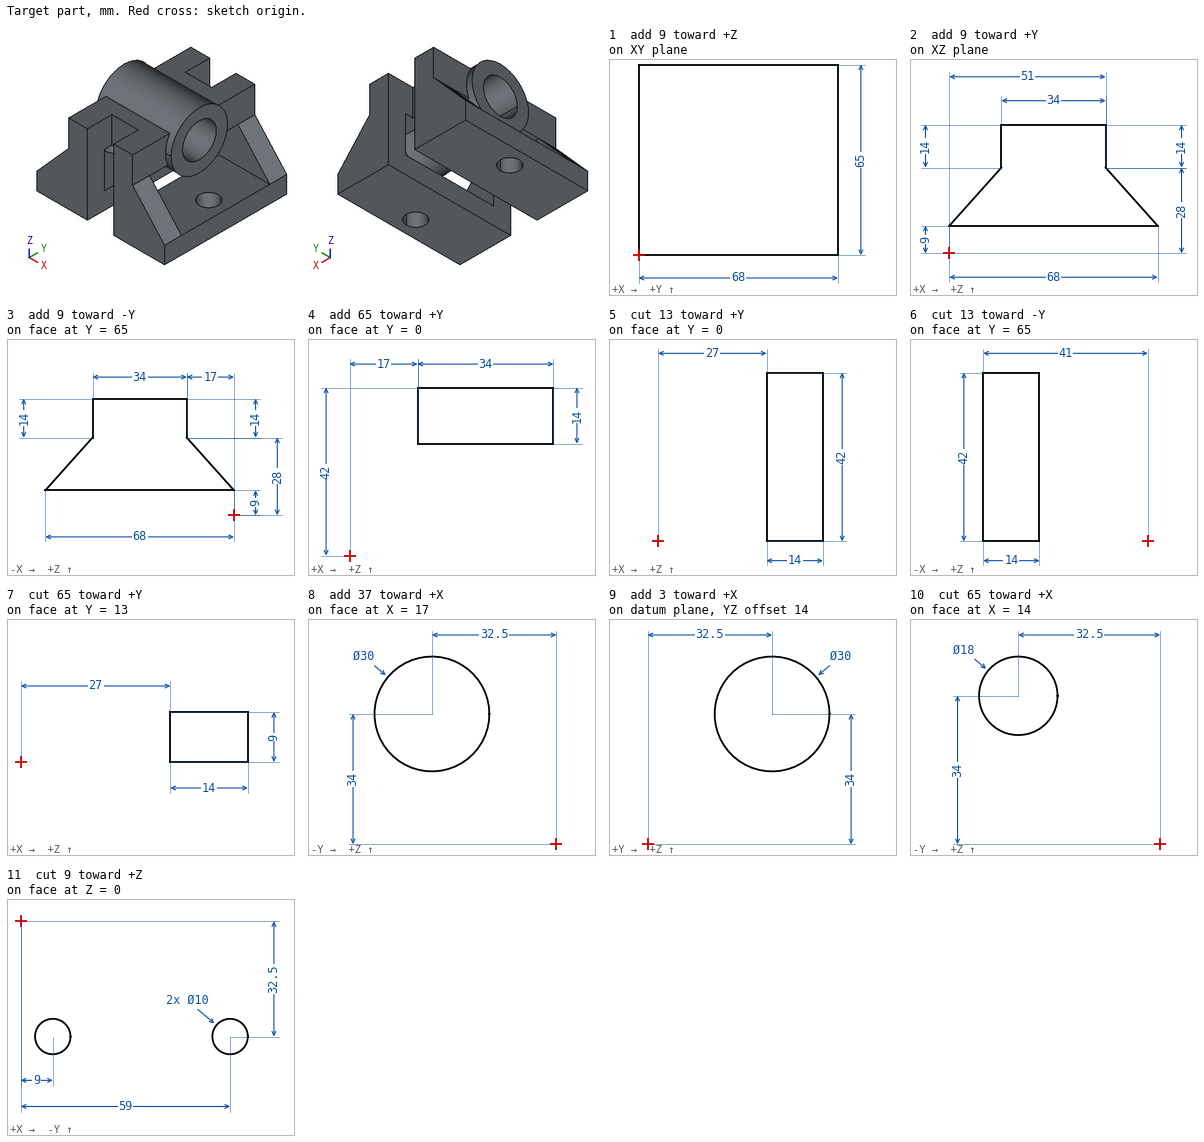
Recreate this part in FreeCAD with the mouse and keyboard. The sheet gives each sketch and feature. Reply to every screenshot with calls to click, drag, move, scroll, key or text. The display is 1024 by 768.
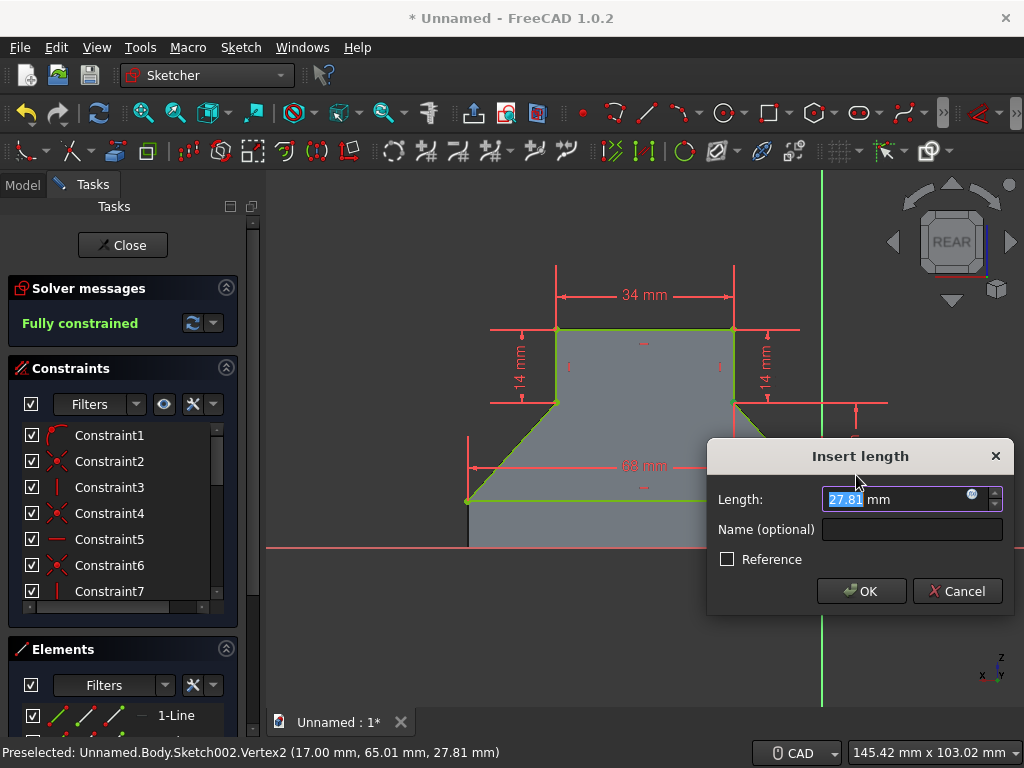
text(28)
key(Return)
key(Escape)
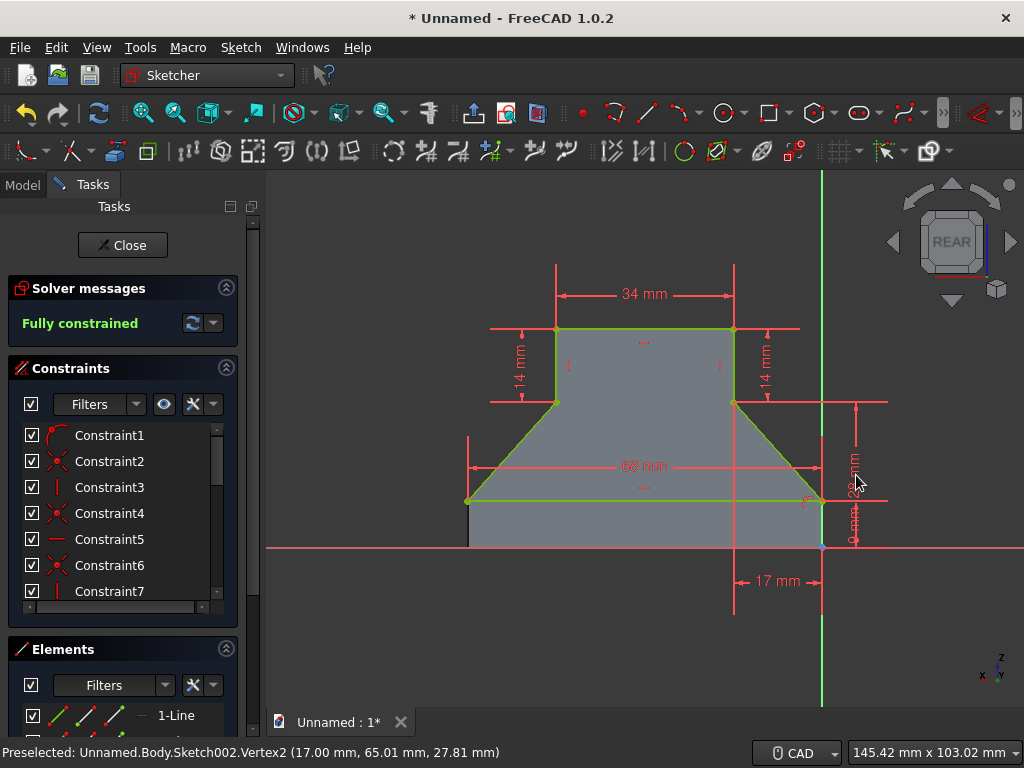
click(123, 245)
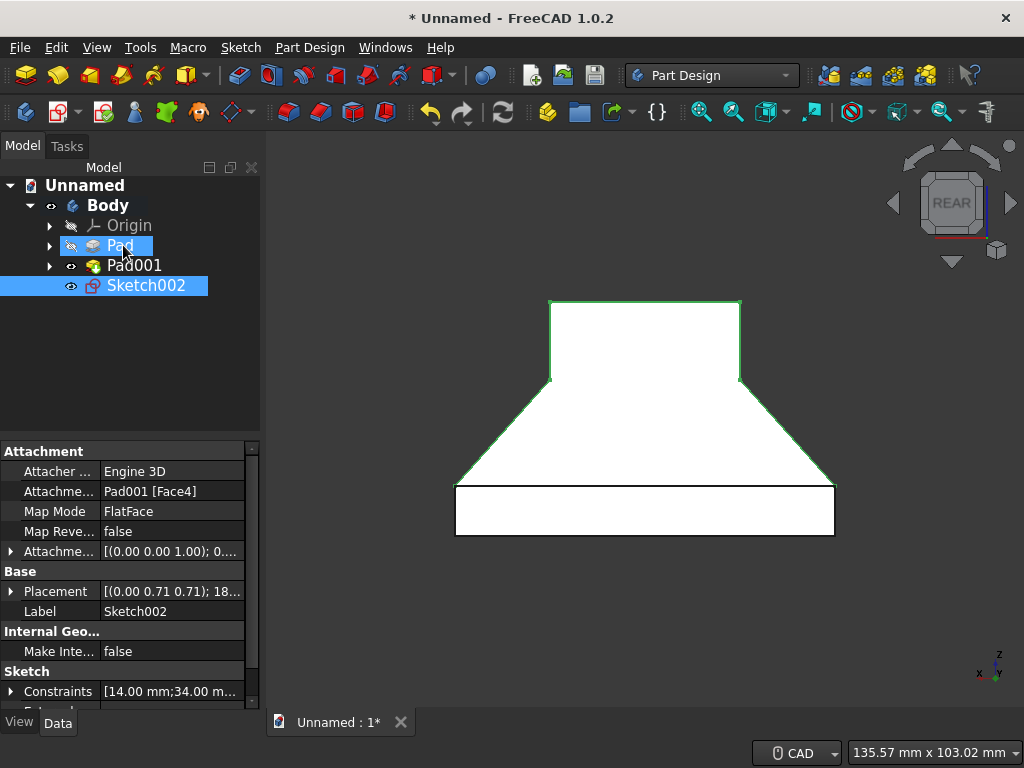
click(26, 76)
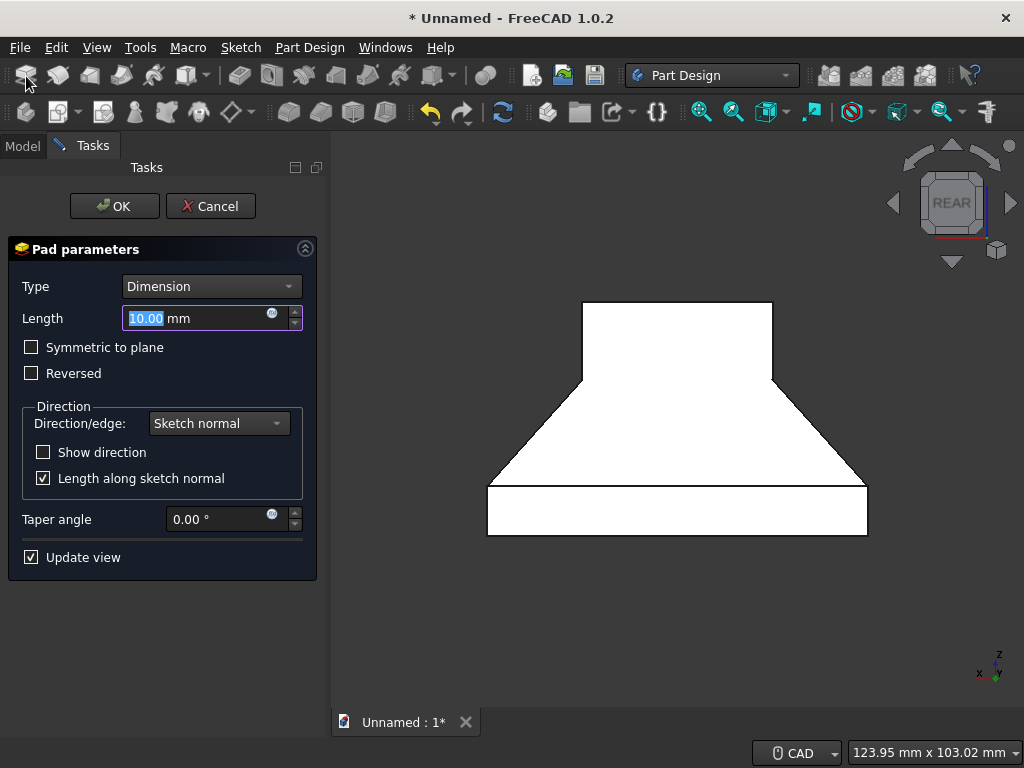
text(9)
key(Tab)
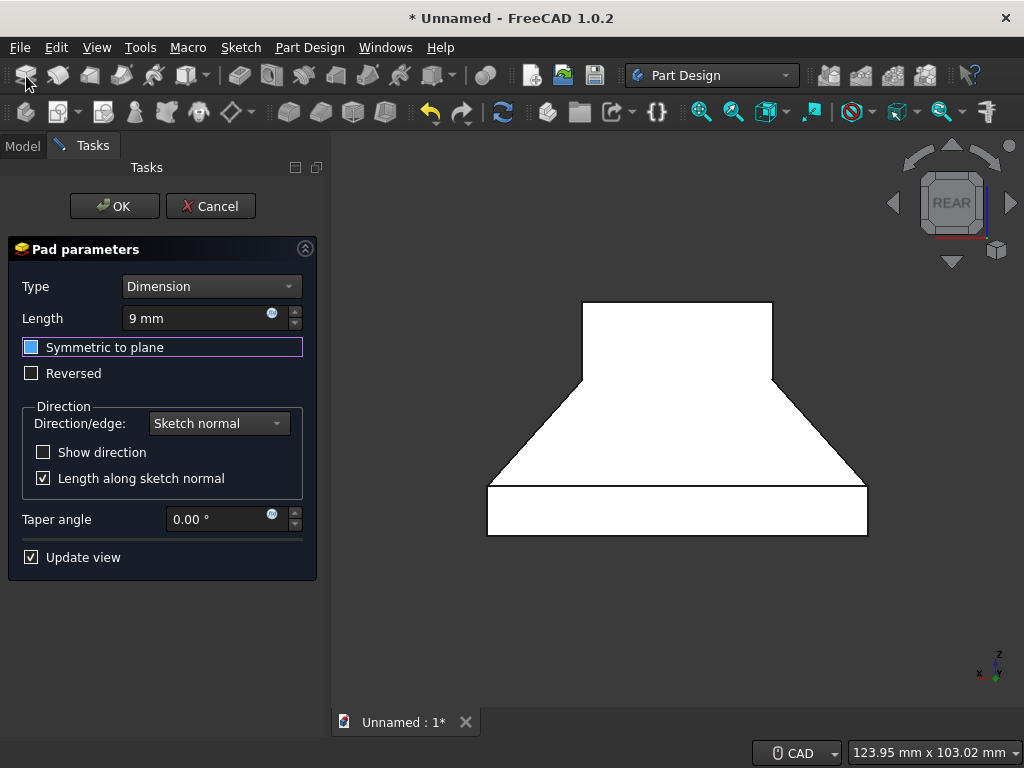
click(30, 373)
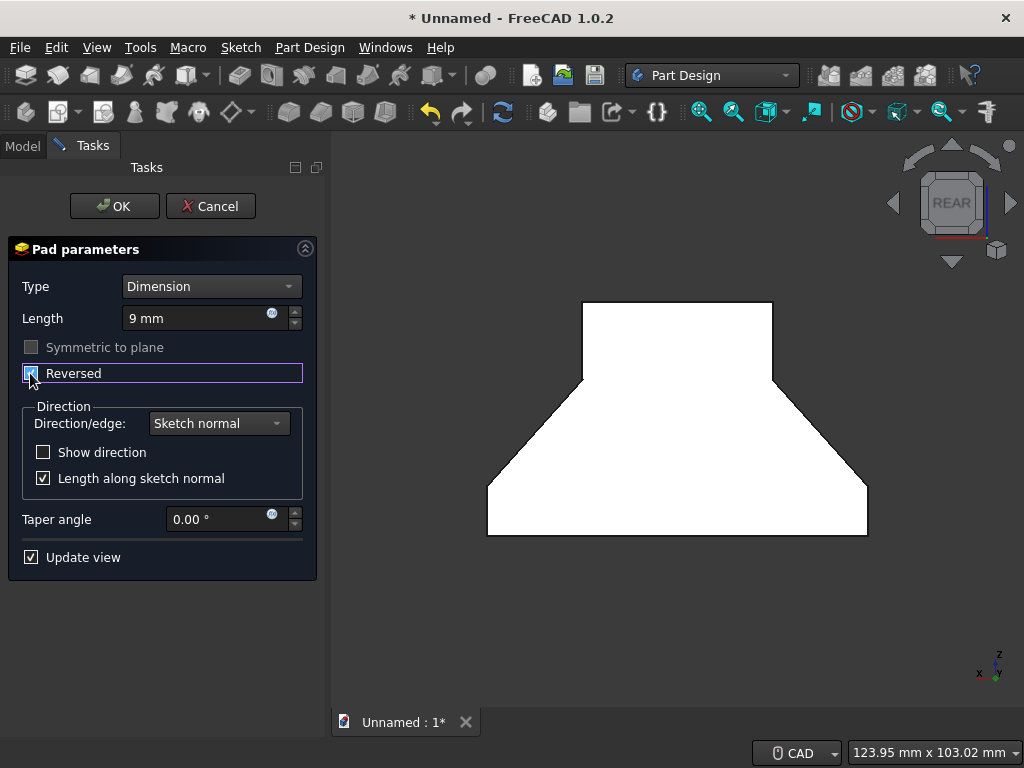
click(115, 206)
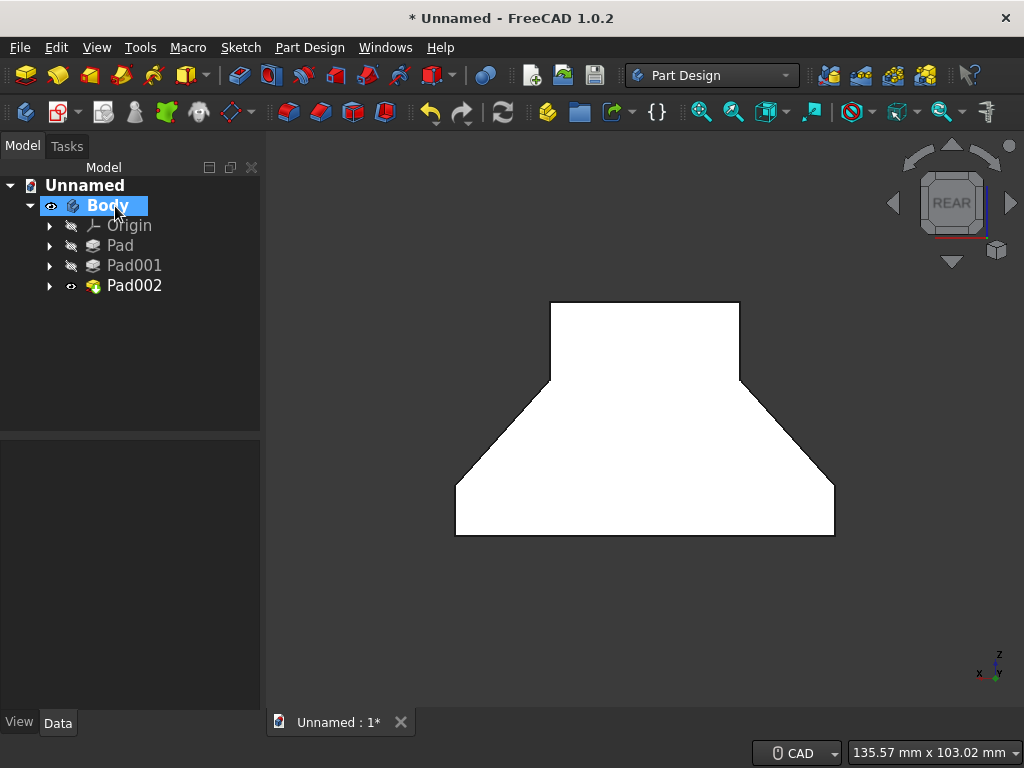
key(0)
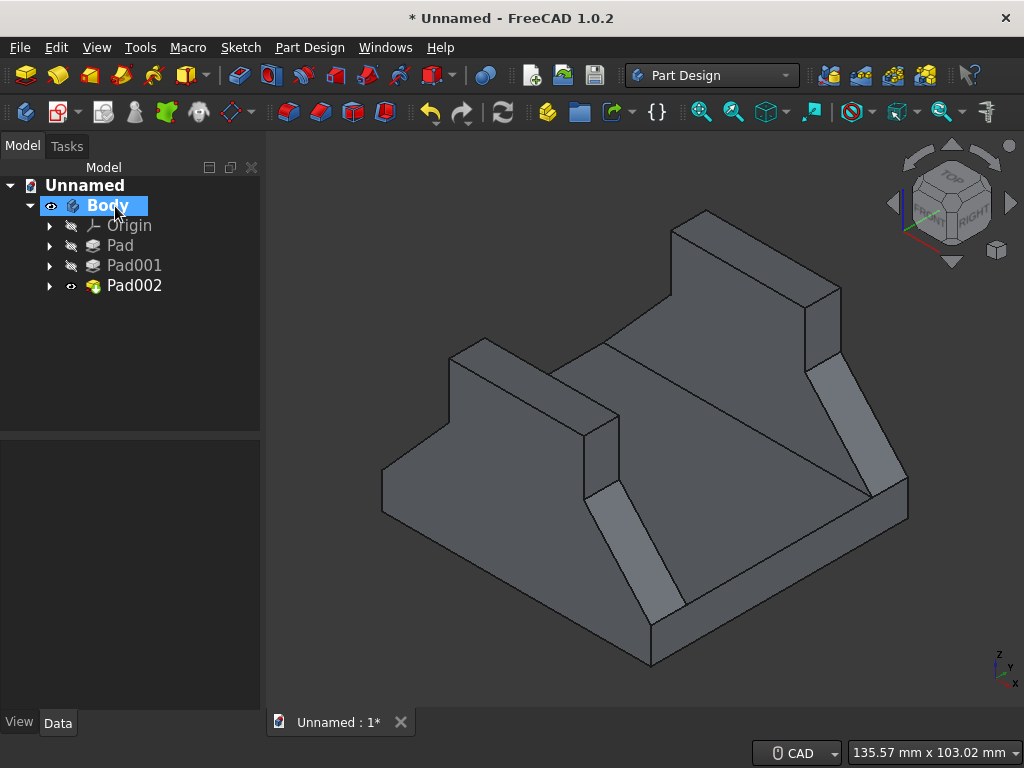
click(517, 492)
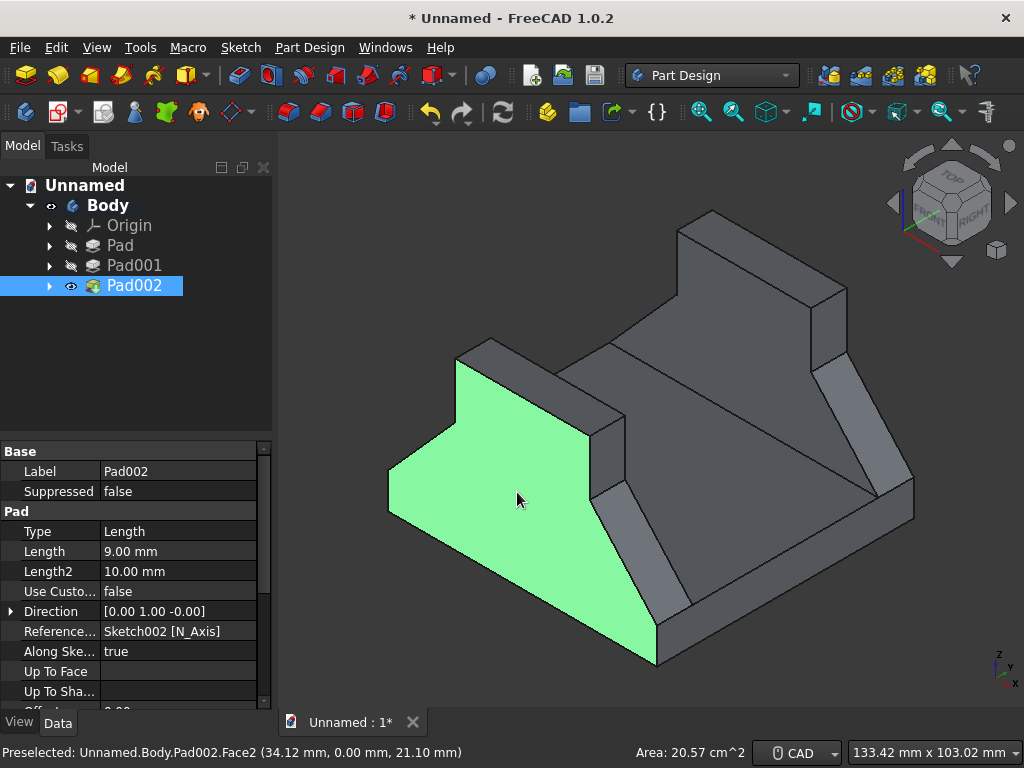
click(58, 112)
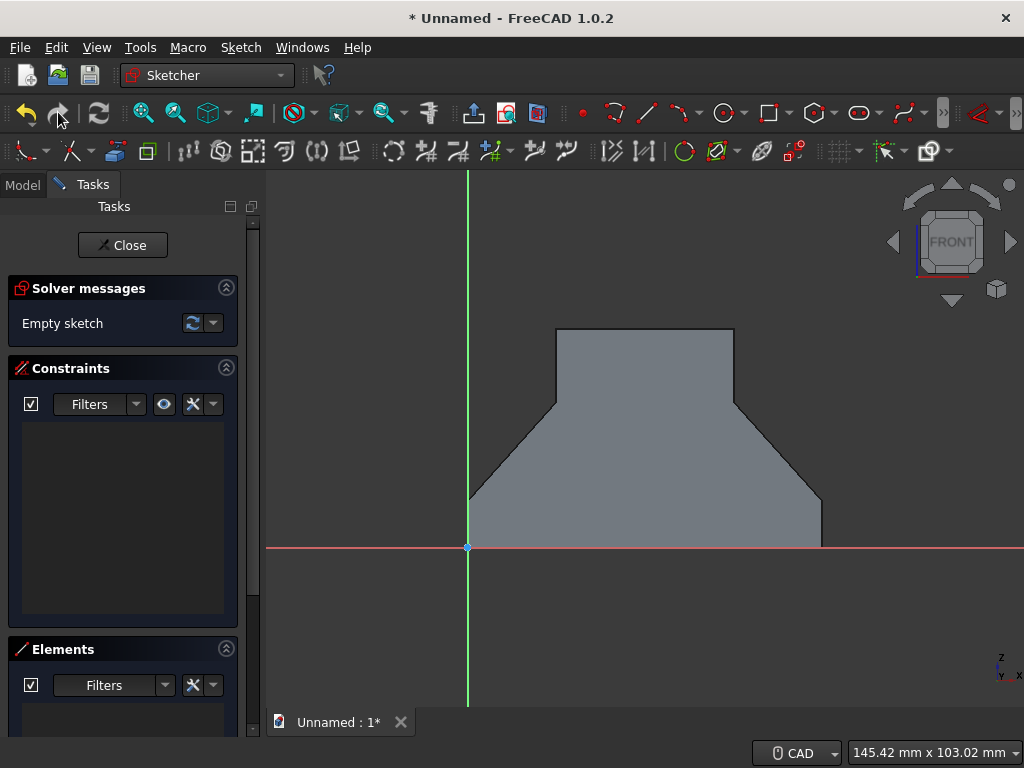
scroll(650, 439, up, 2)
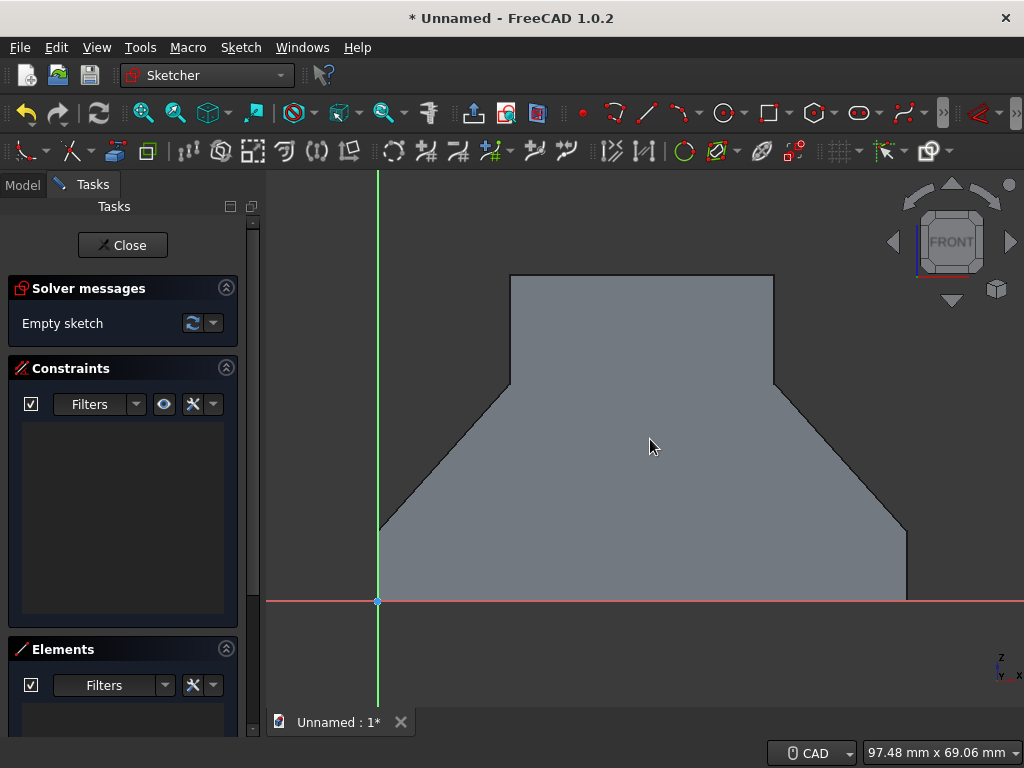
click(770, 114)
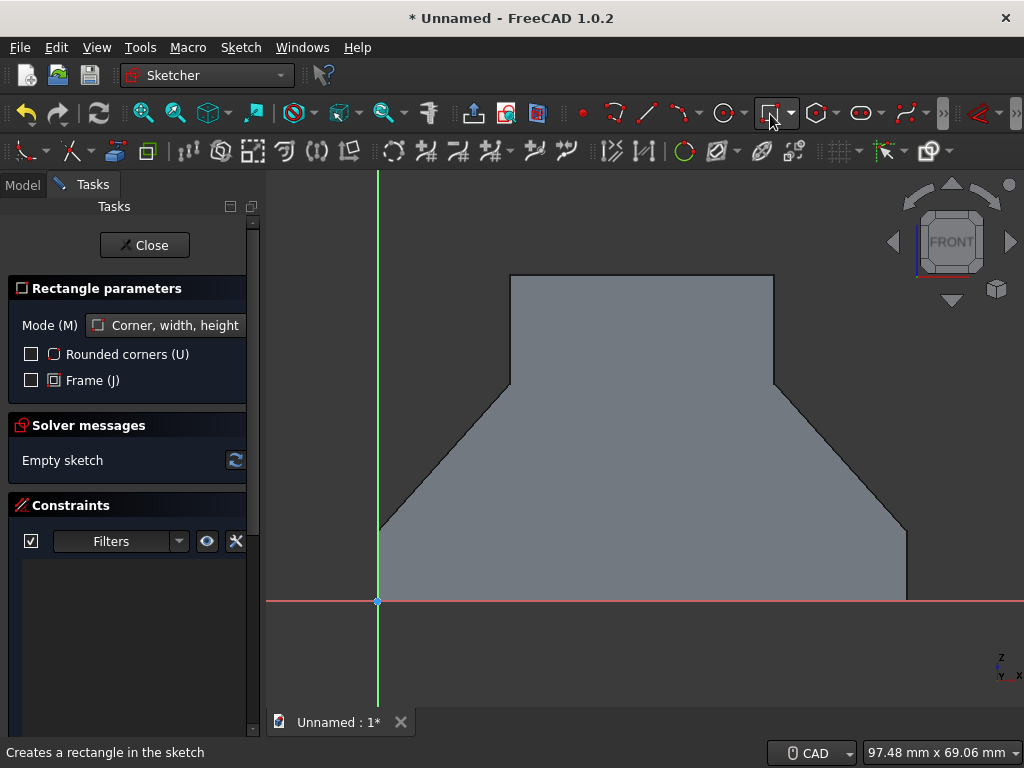
click(510, 275)
move(774, 384)